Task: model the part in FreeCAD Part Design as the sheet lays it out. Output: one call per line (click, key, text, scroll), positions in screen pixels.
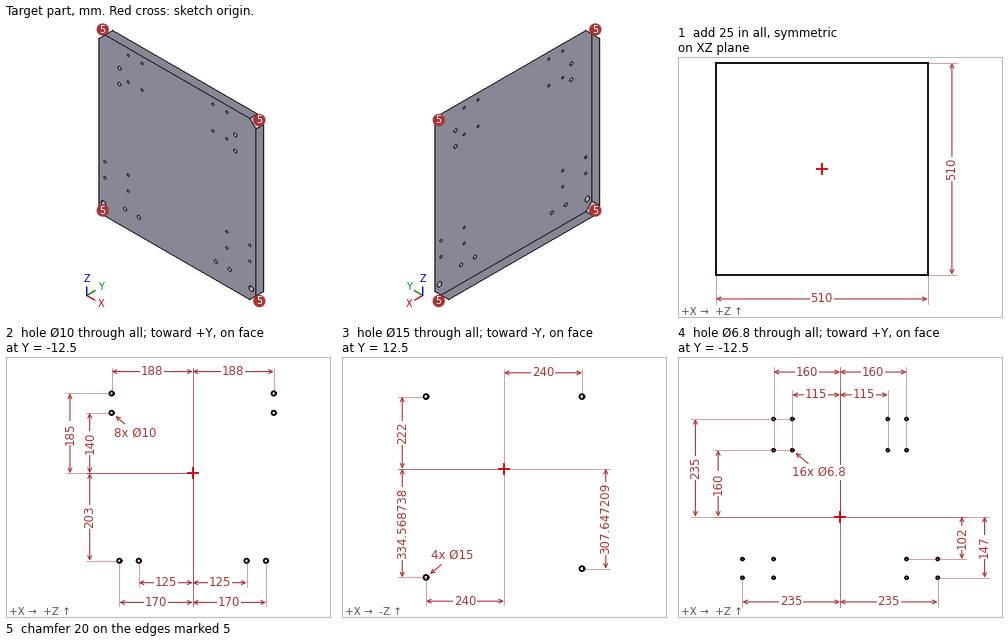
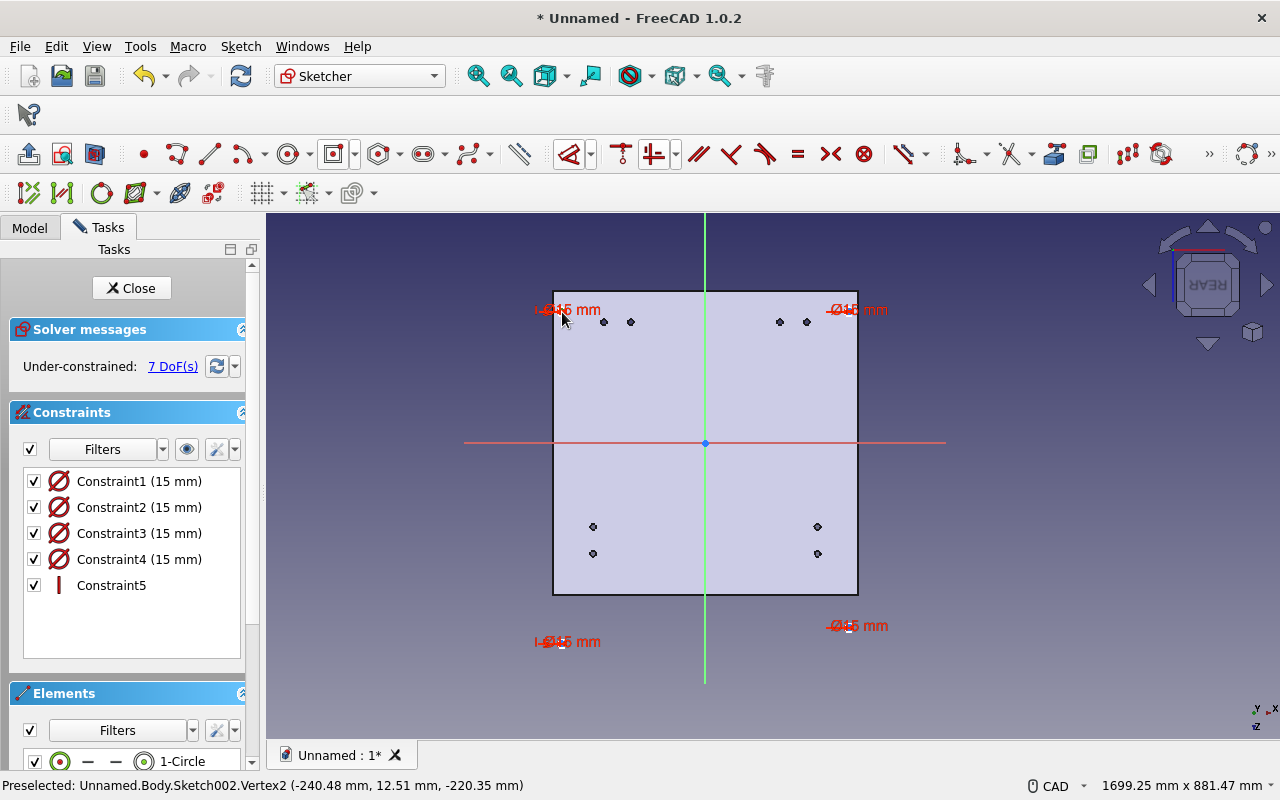
click(849, 312)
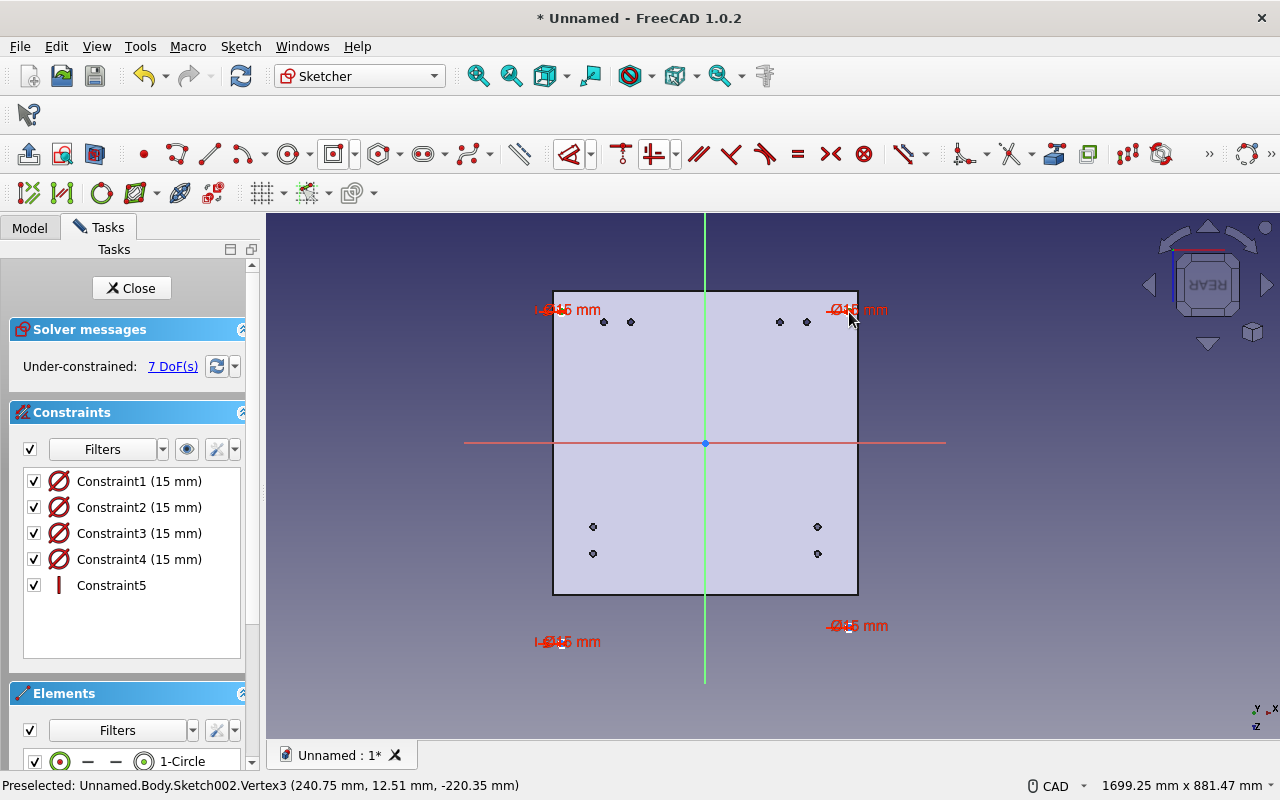
click(676, 154)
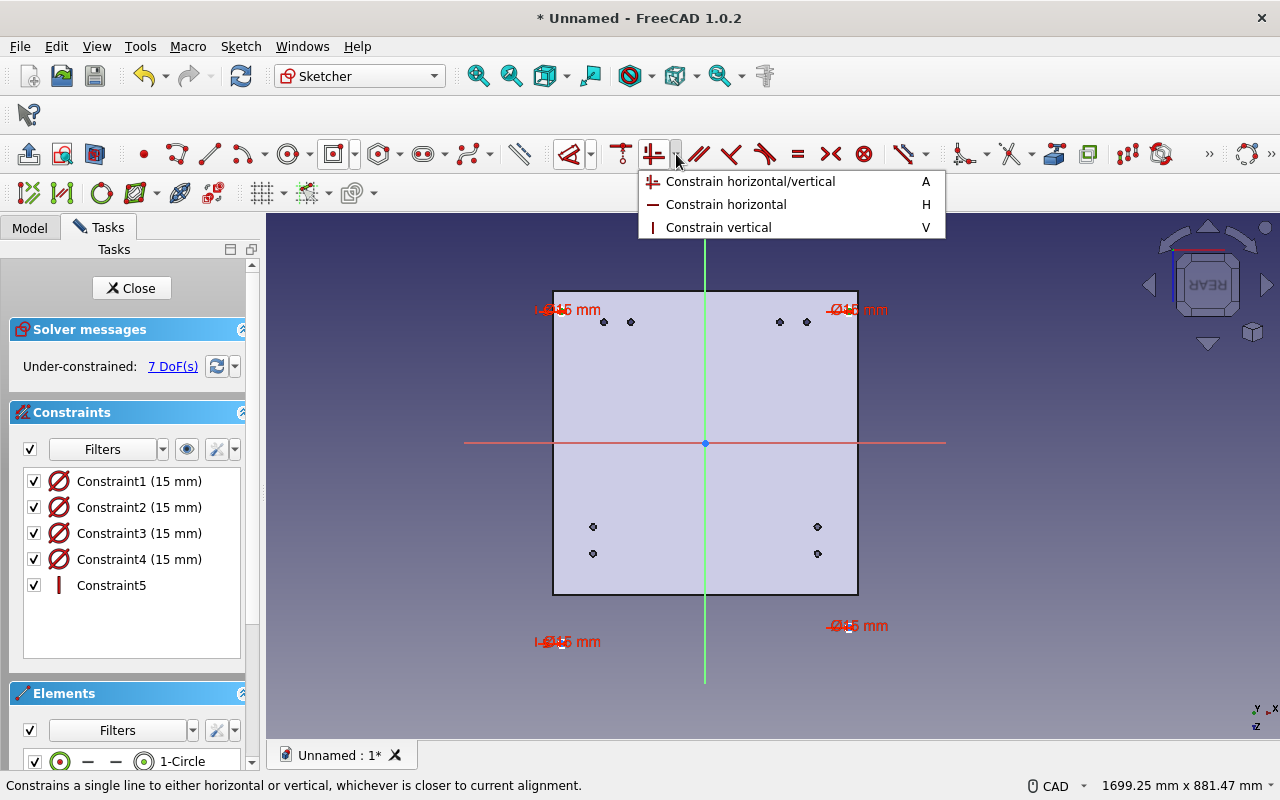
click(792, 204)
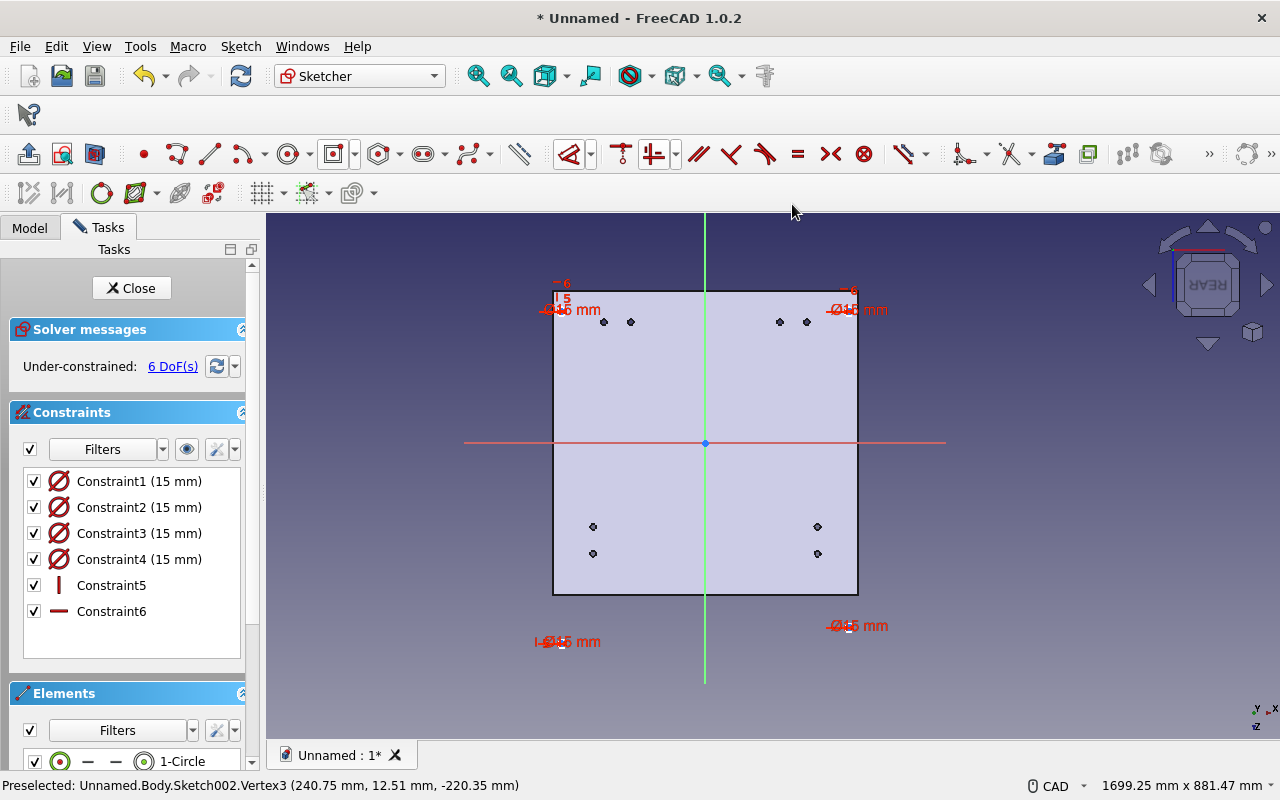
click(849, 312)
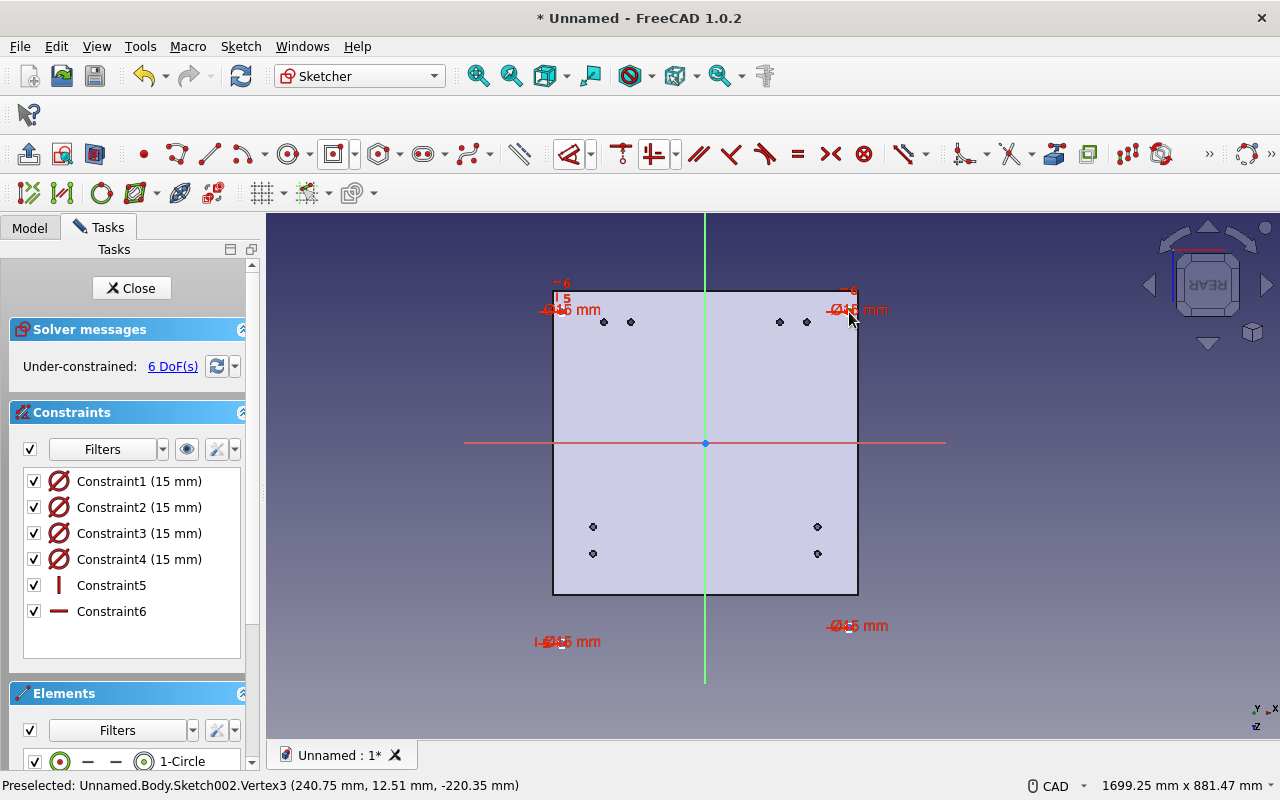
click(849, 628)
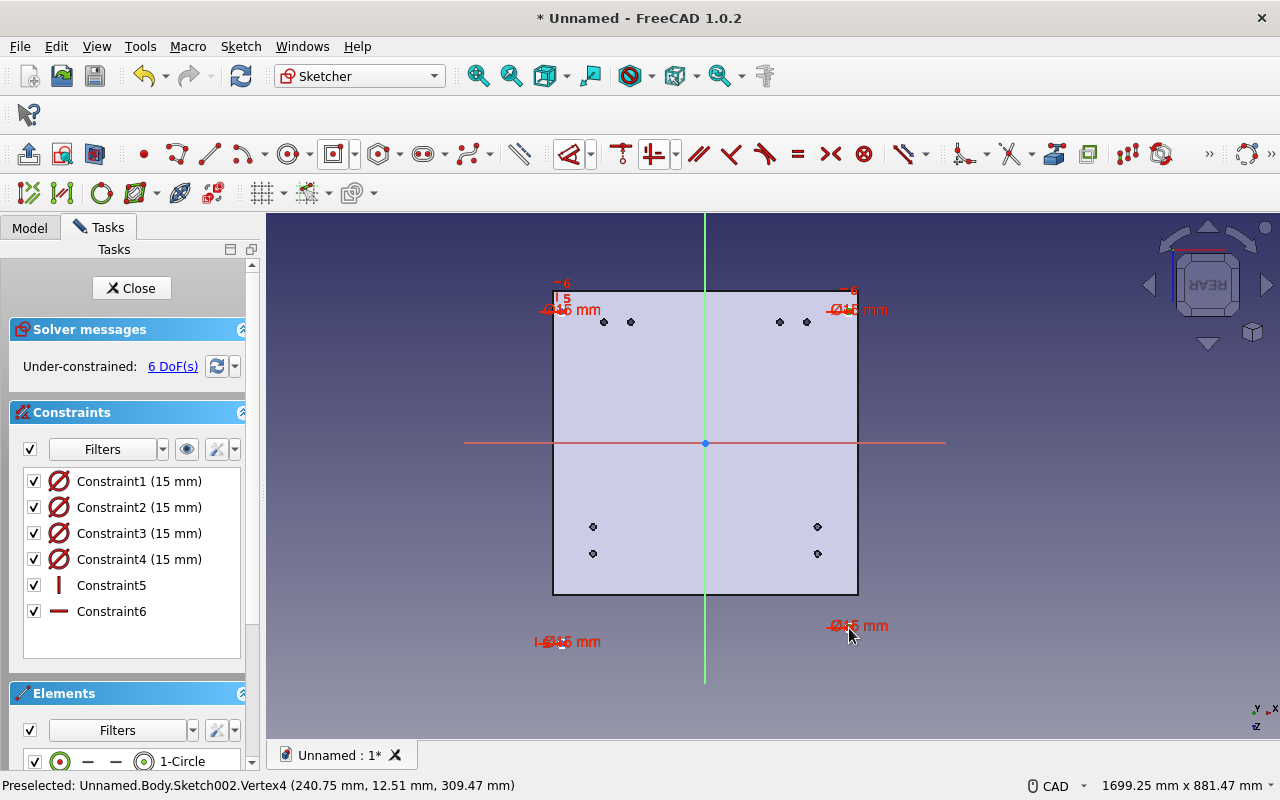
click(676, 154)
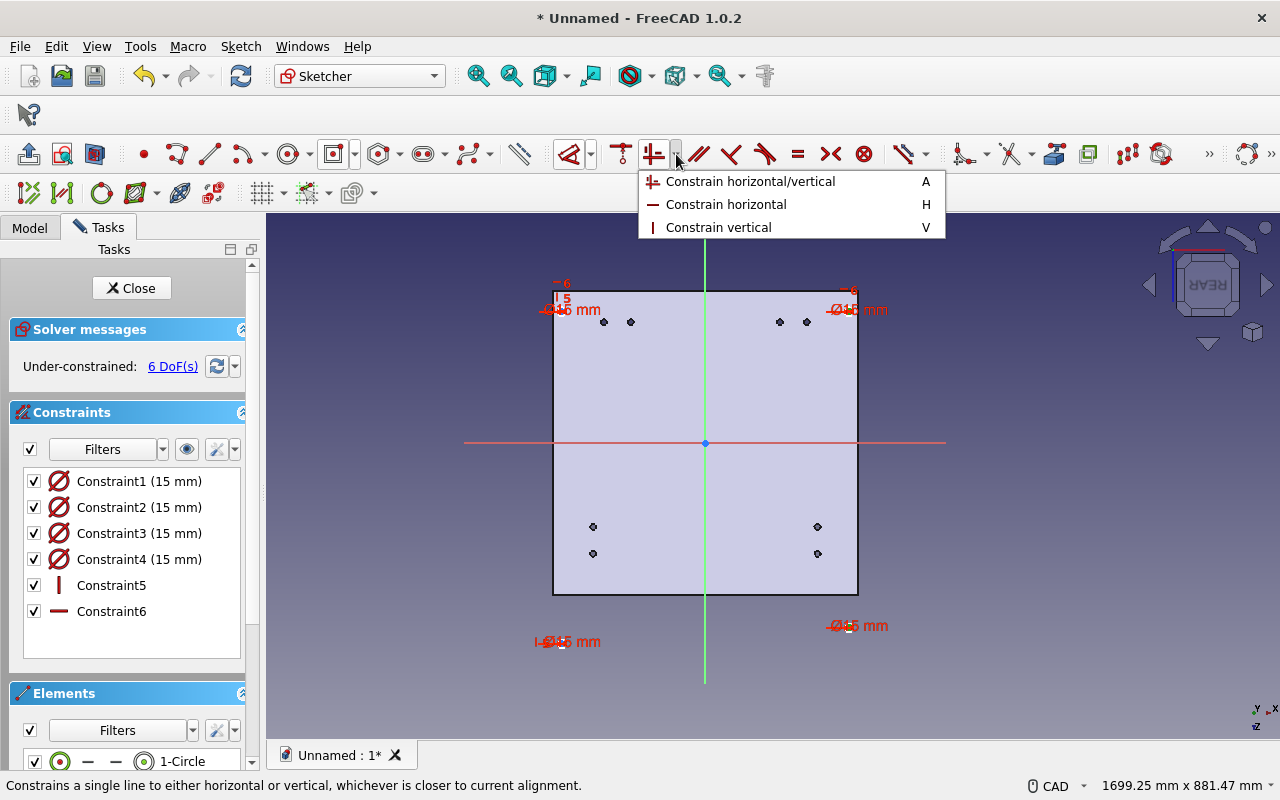
click(792, 228)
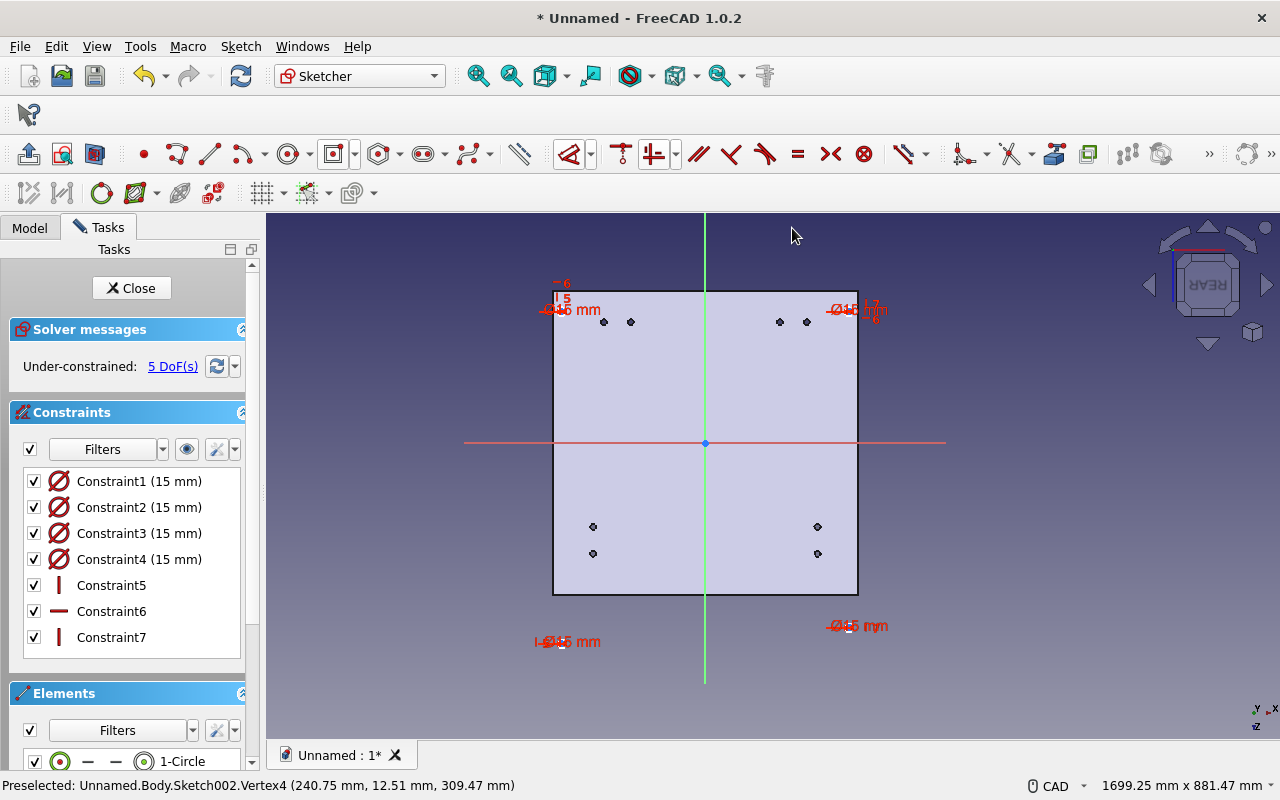
click(562, 644)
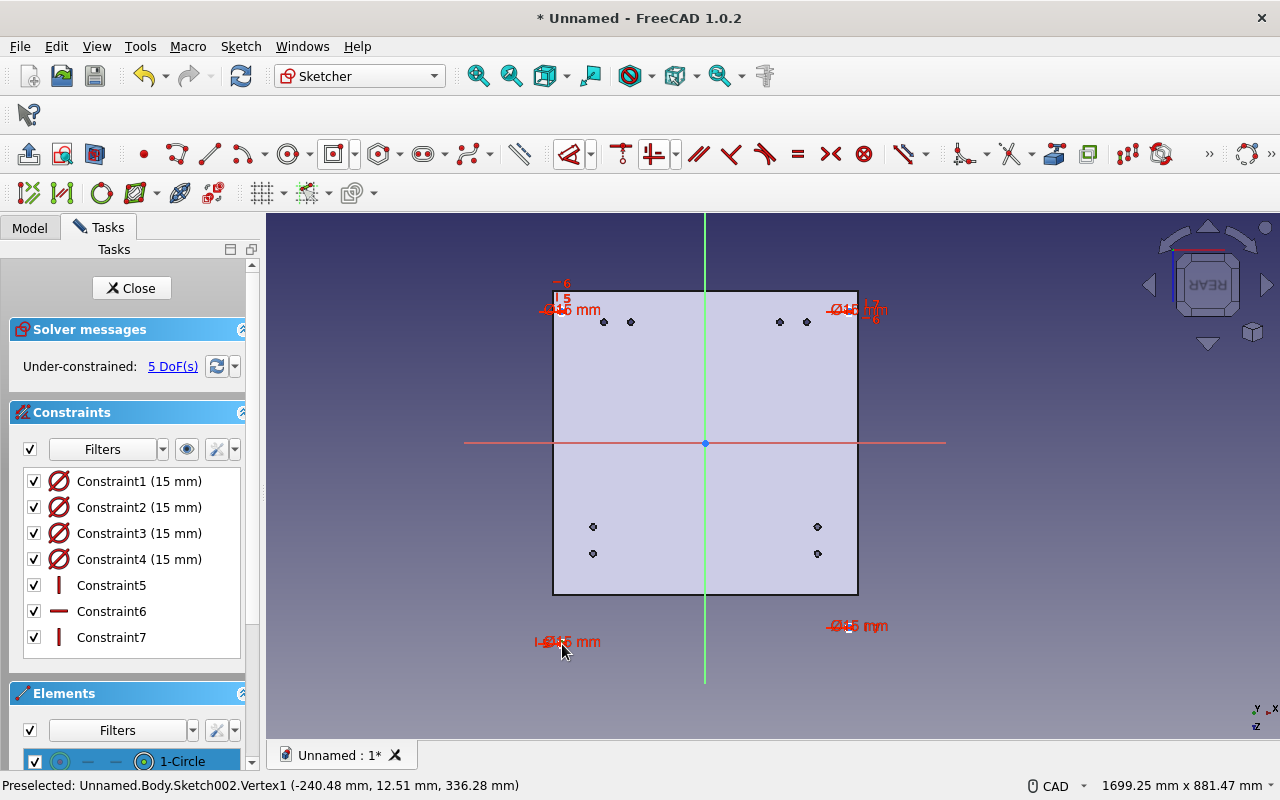
key(l)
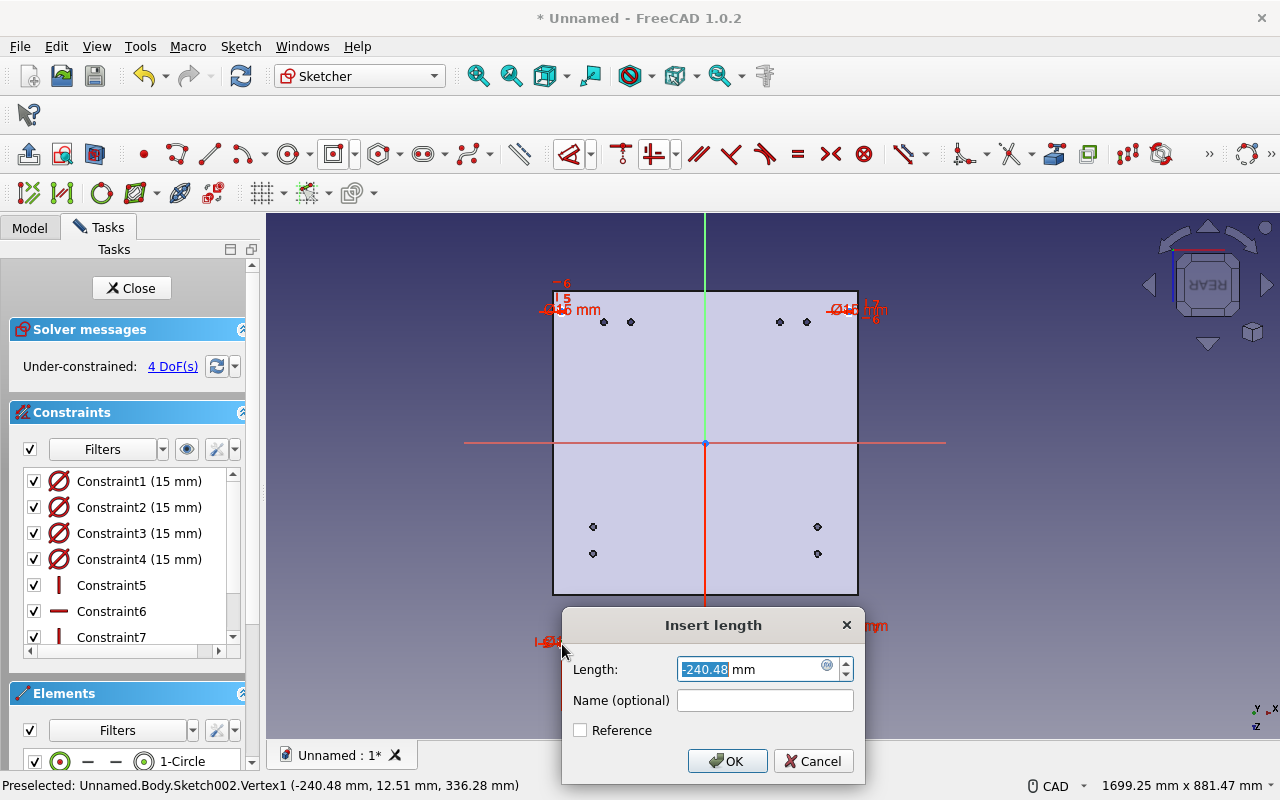
text(-240)
key(Return)